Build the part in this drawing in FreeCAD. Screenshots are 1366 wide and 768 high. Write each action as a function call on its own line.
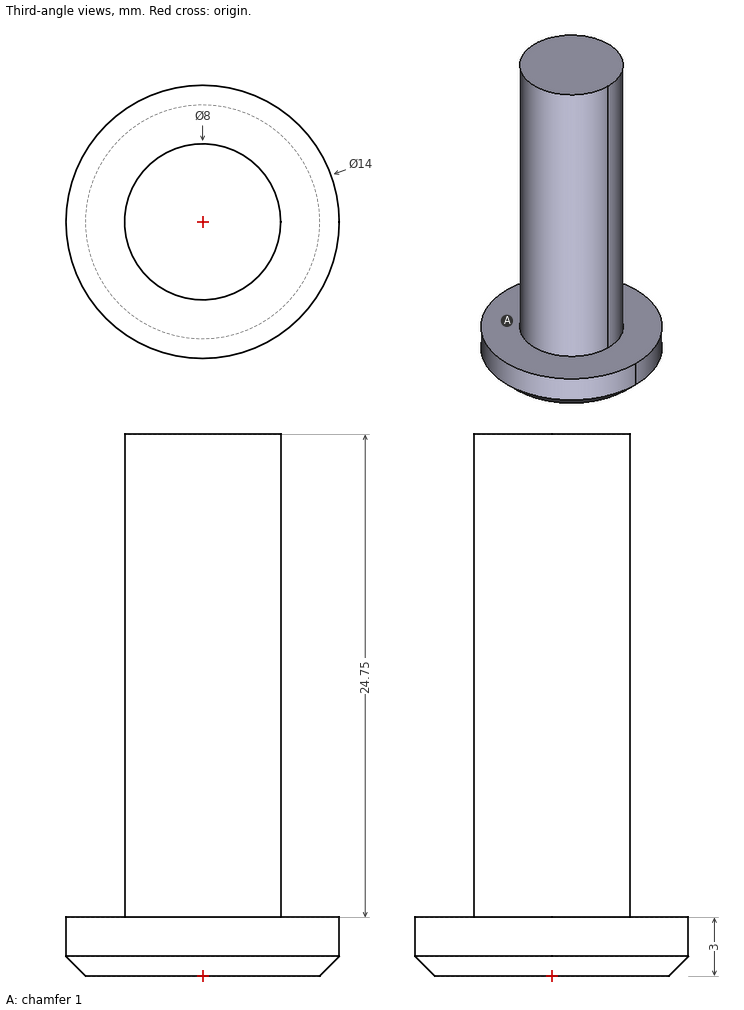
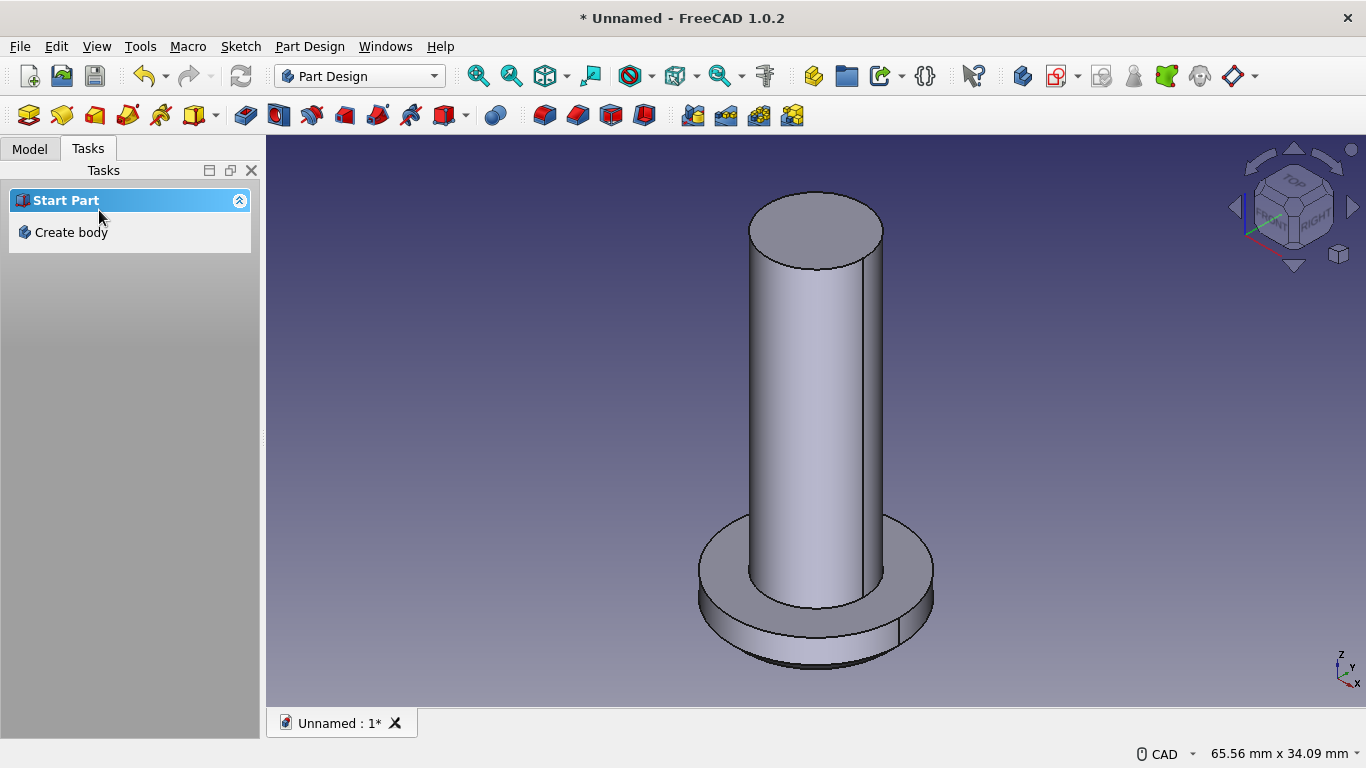
click(479, 76)